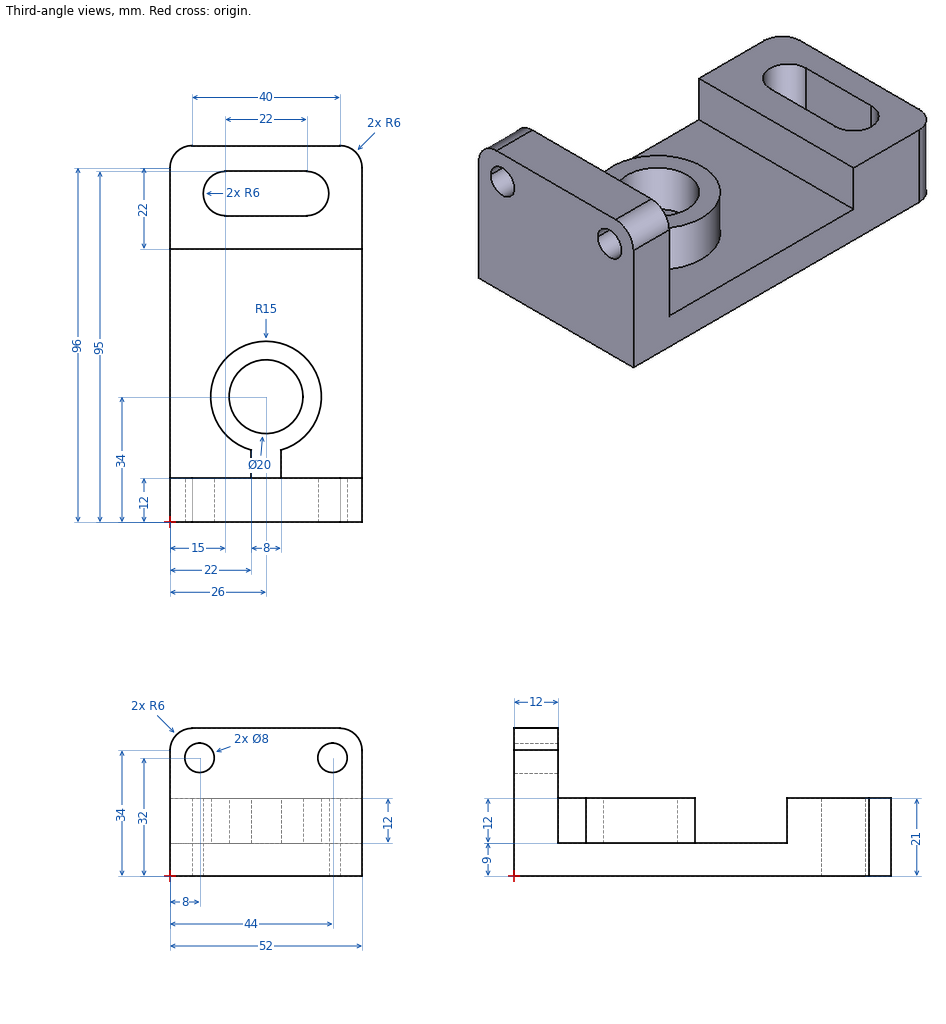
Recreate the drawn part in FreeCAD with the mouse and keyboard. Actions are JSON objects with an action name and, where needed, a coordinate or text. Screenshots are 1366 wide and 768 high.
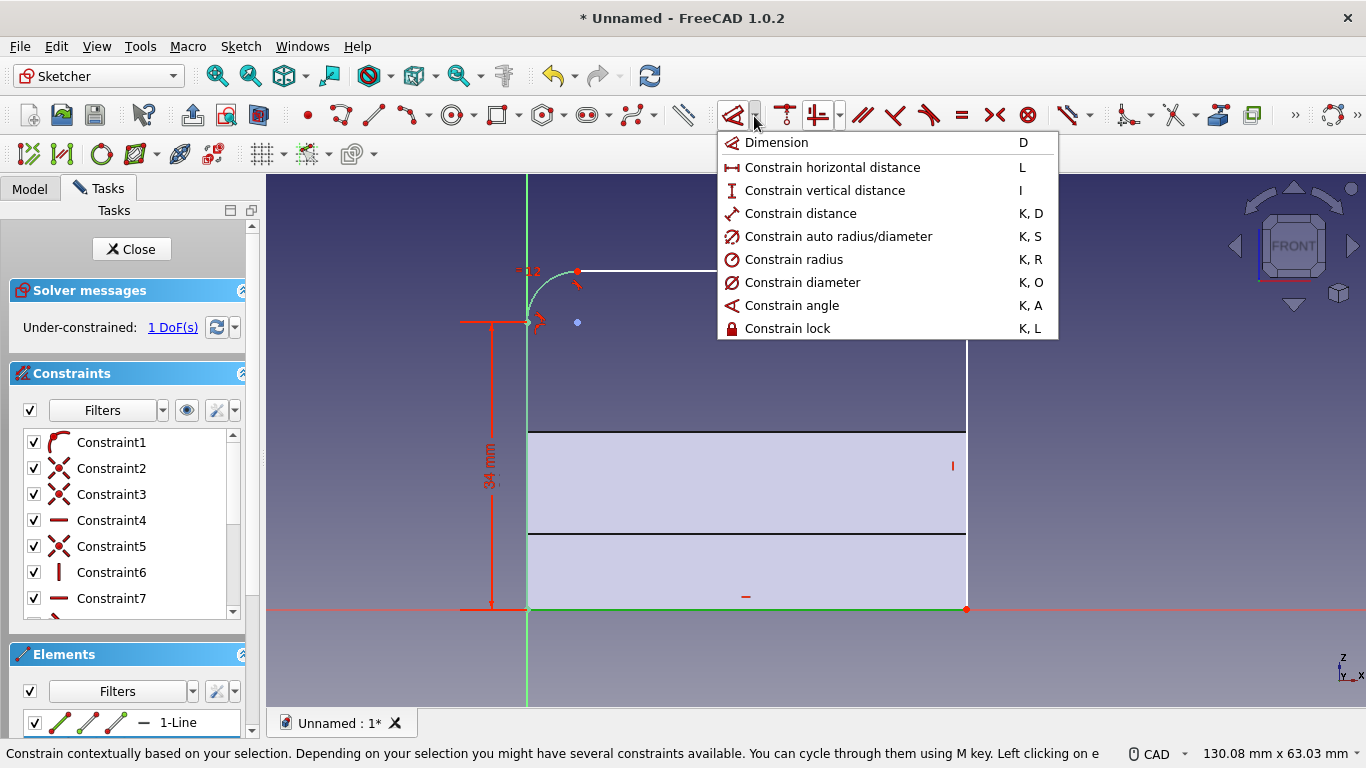
{"action": "left_click", "coordinate": [888, 168]}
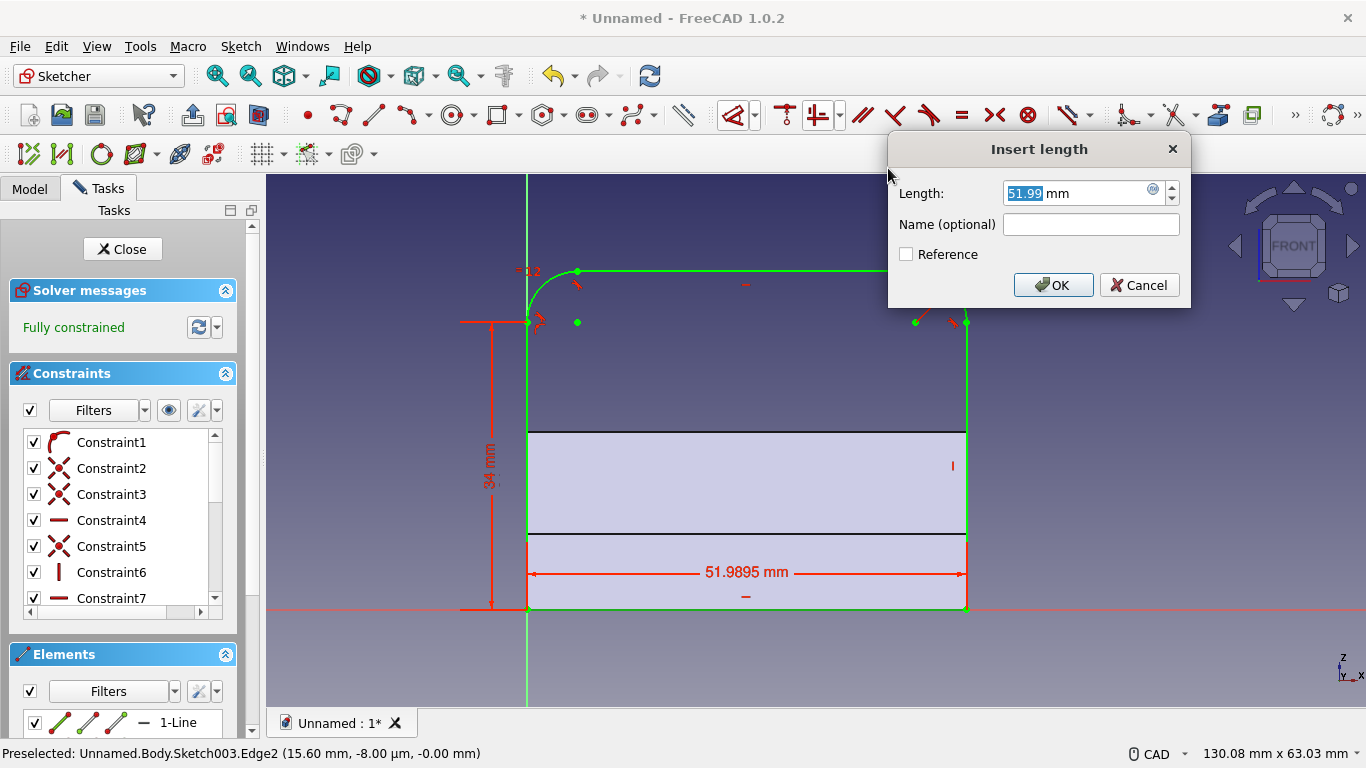
{"action": "type", "text": "52"}
{"action": "key", "text": "Return"}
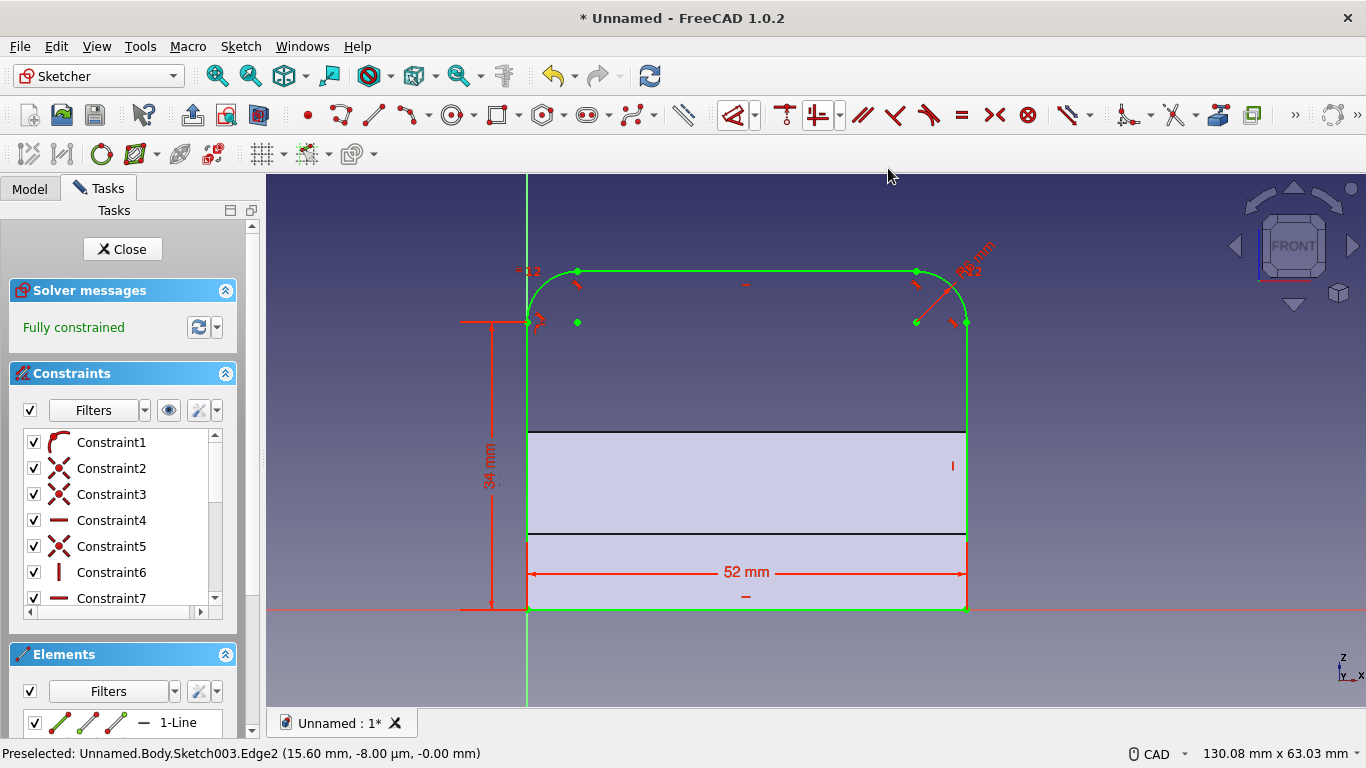
{"action": "left_click", "coordinate": [123, 249]}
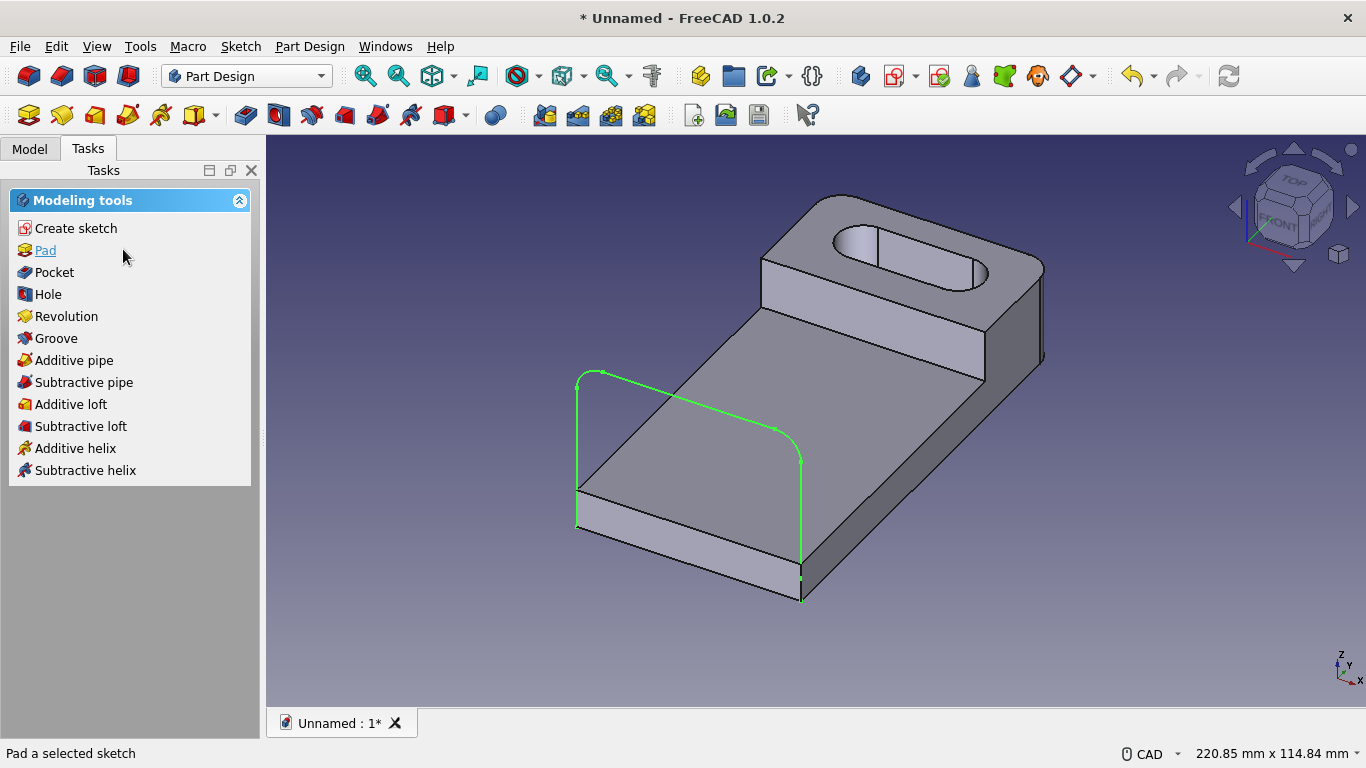
{"action": "left_click", "coordinate": [29, 116]}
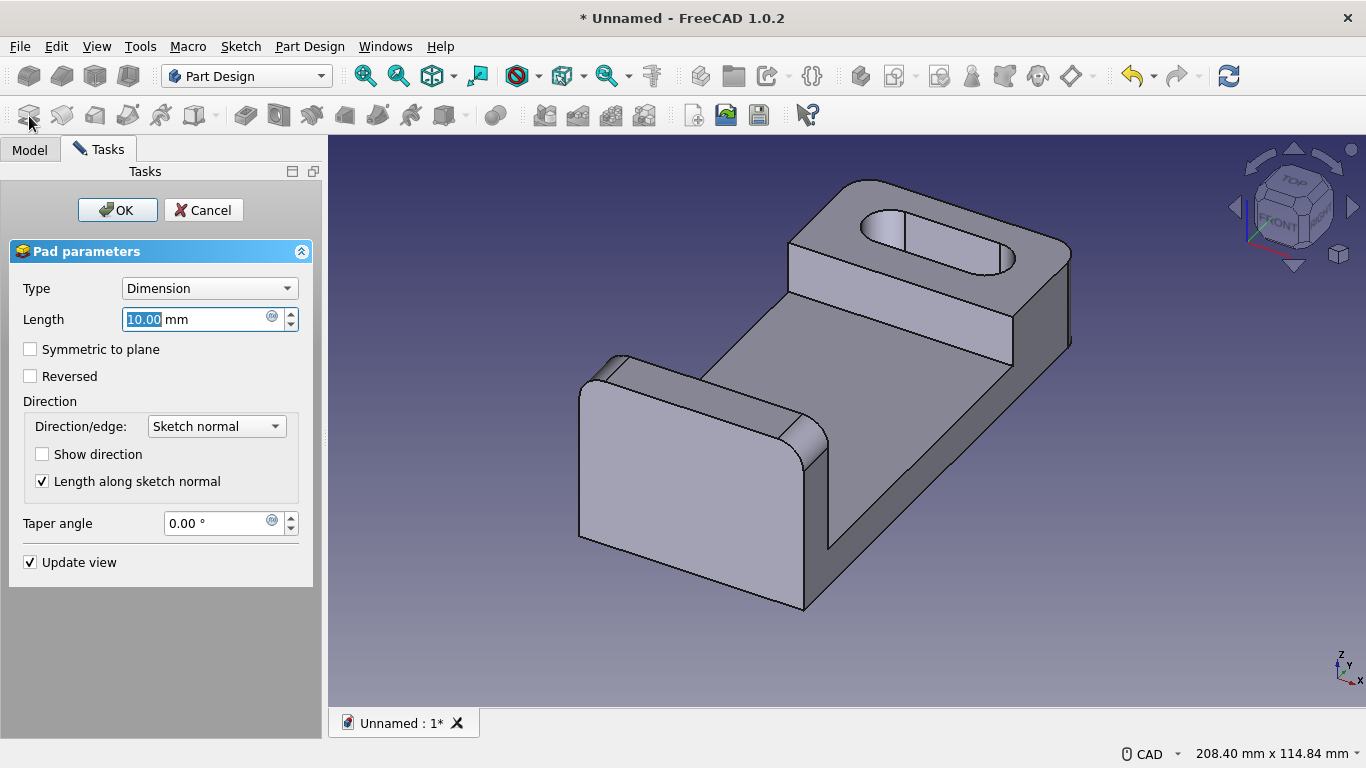
{"action": "type", "text": "12"}
{"action": "key", "text": "Tab"}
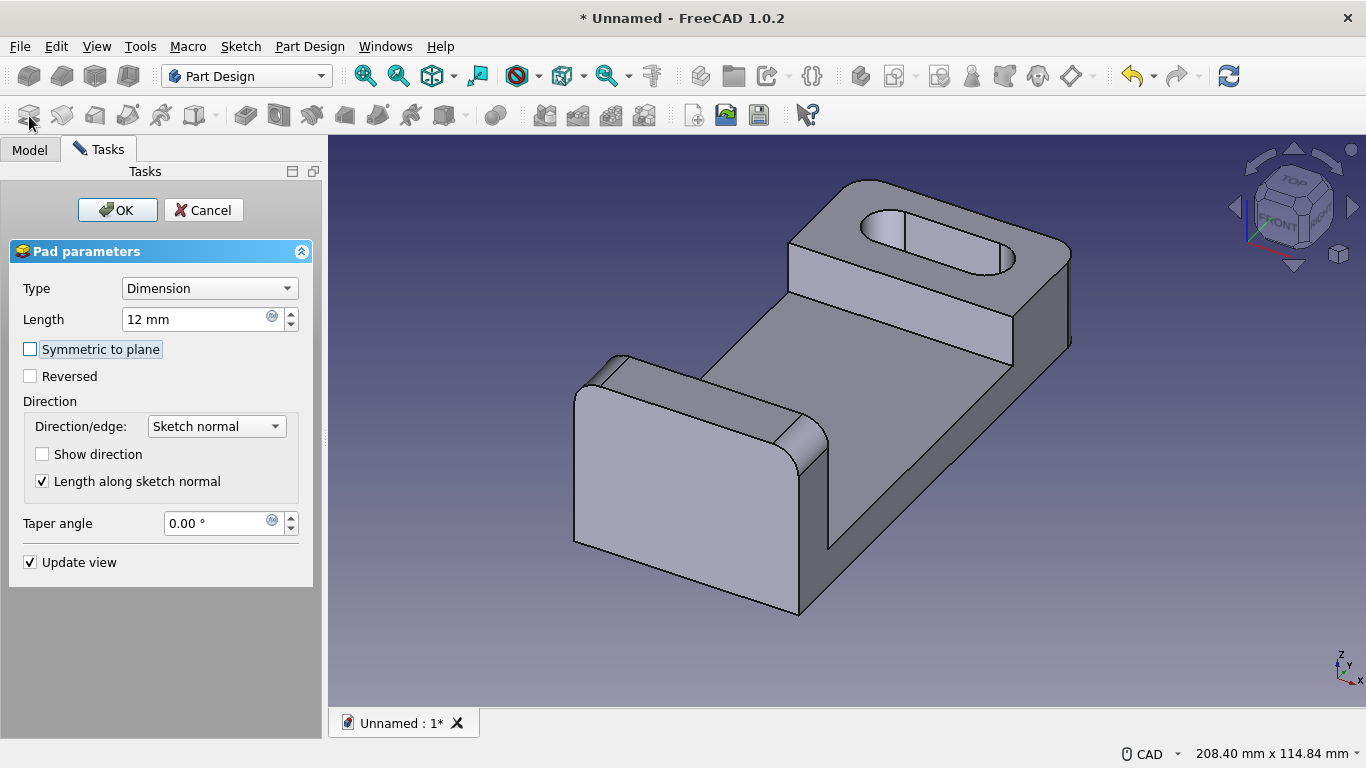
{"action": "left_click", "coordinate": [31, 376]}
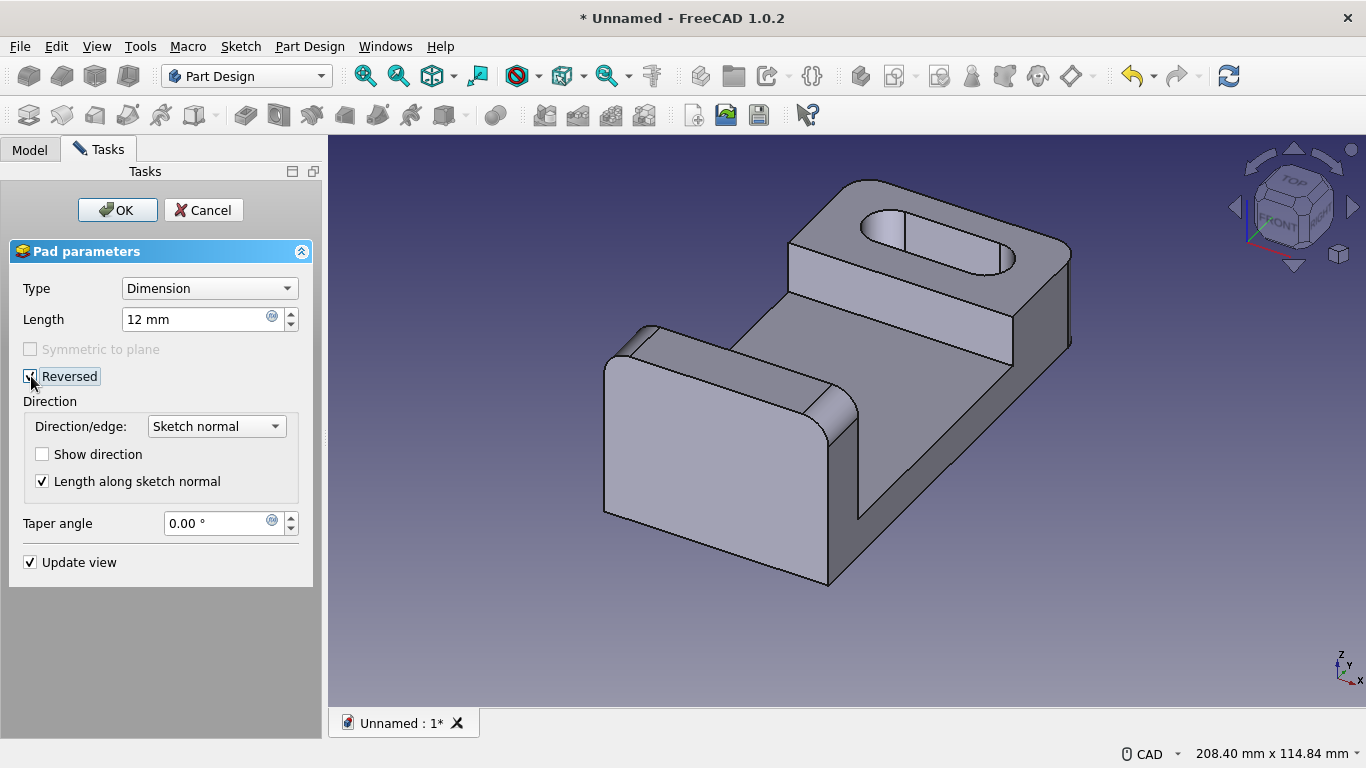
{"action": "left_click", "coordinate": [118, 210]}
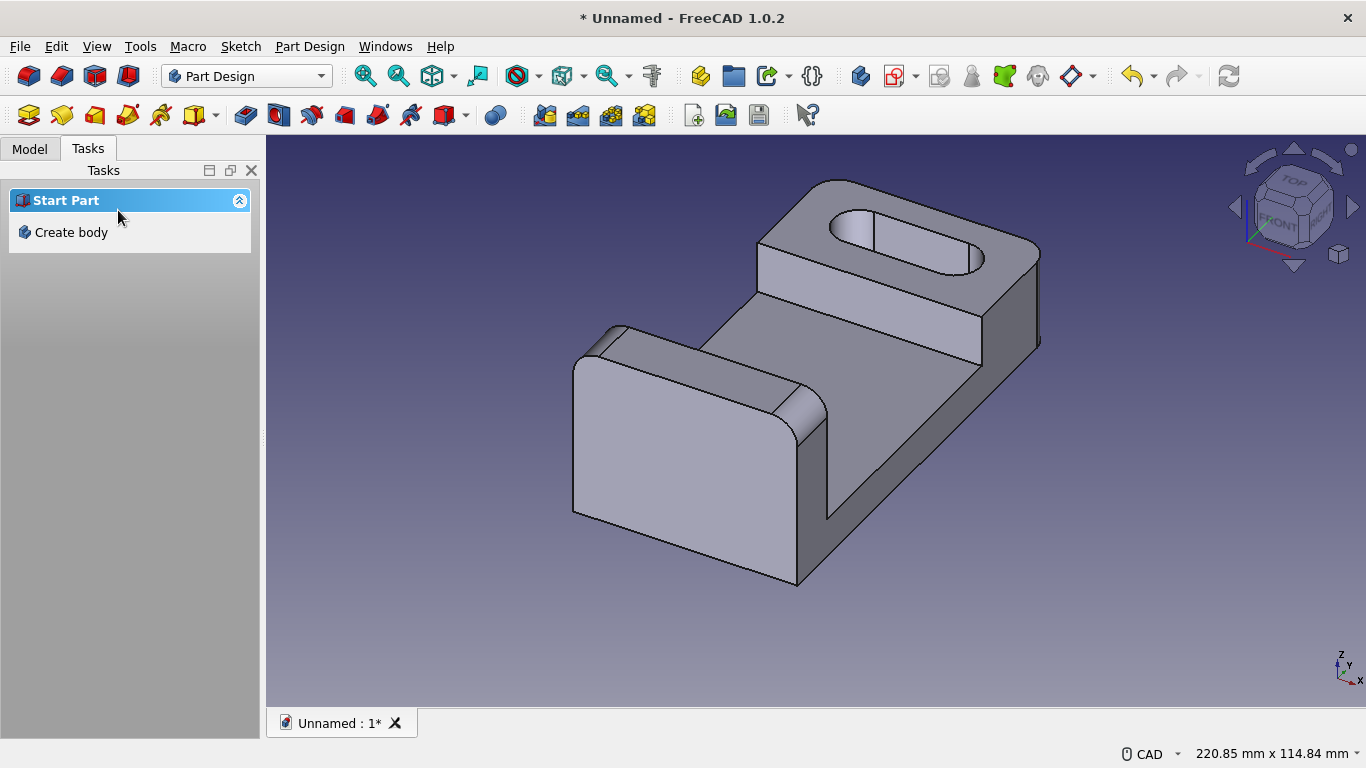
{"action": "left_click", "coordinate": [366, 76]}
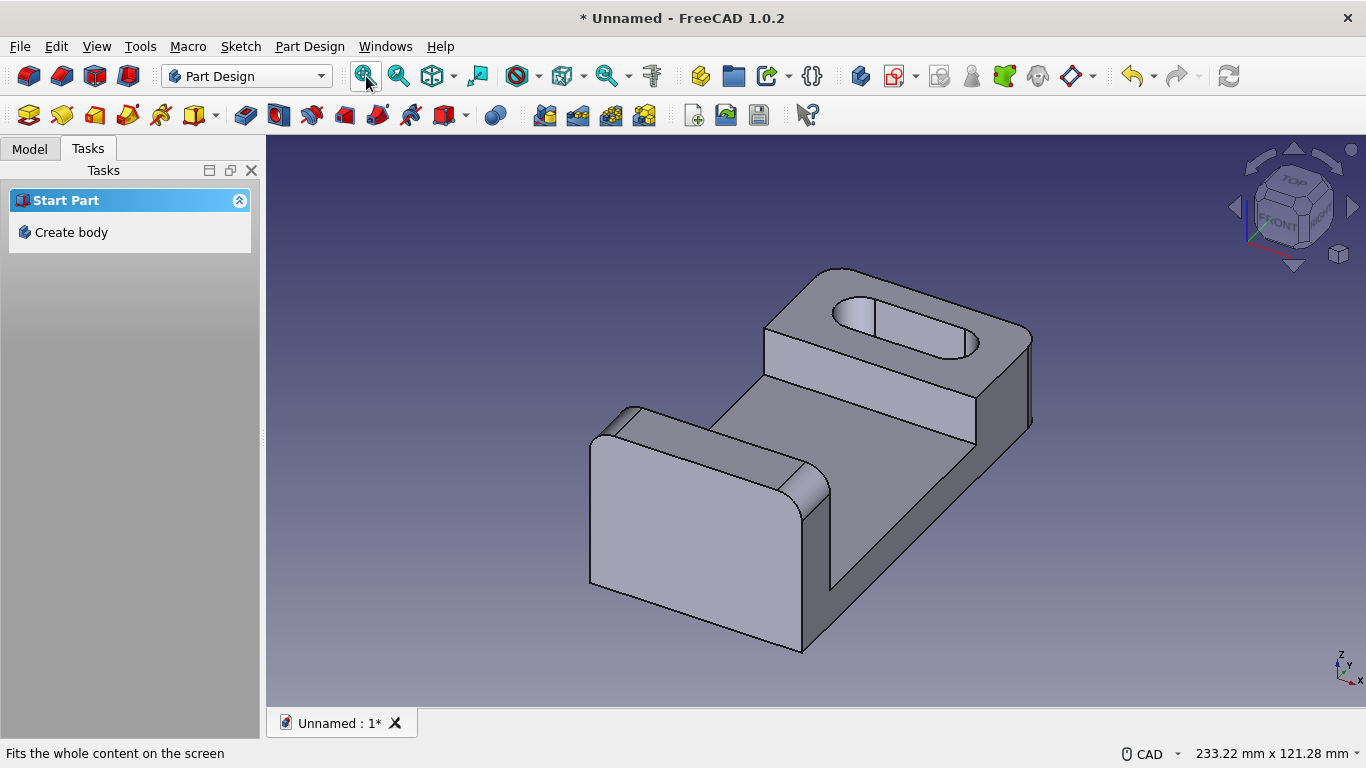
{"action": "key", "text": "4"}